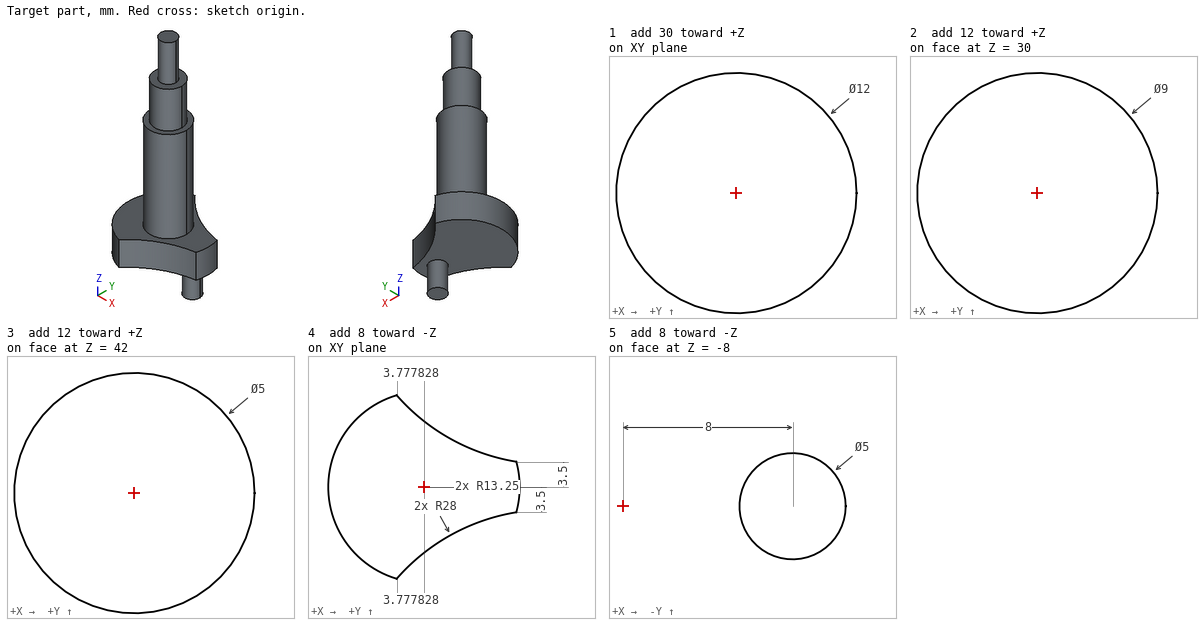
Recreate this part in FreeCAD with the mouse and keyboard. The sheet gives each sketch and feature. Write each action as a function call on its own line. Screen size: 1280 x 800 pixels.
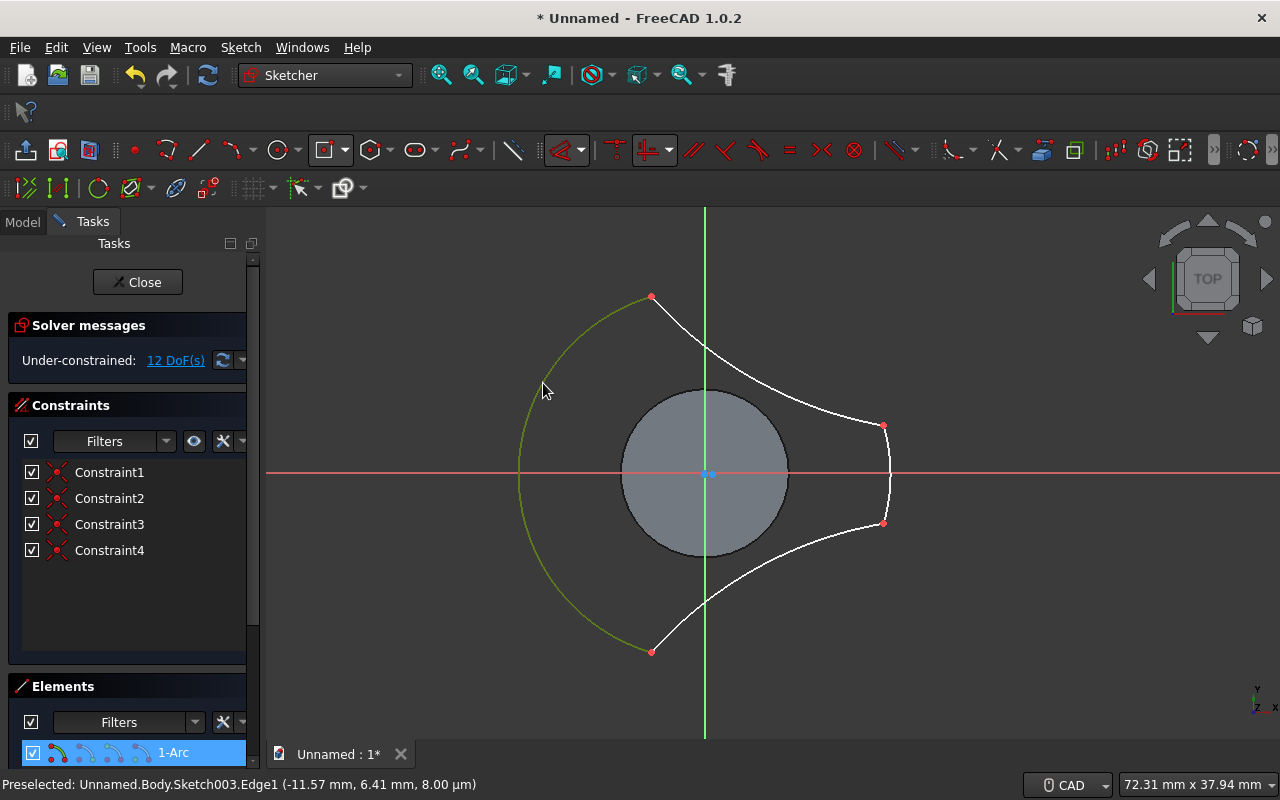
click(889, 494)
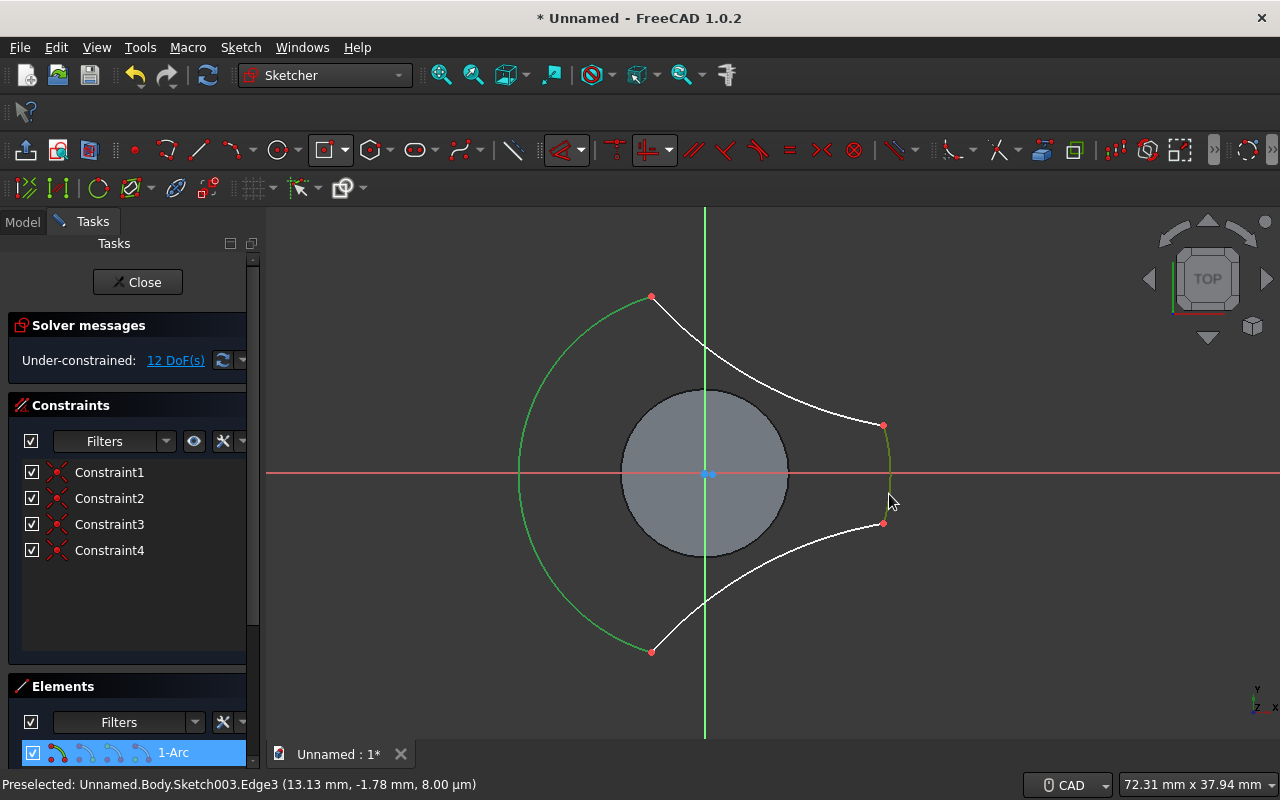
click(616, 150)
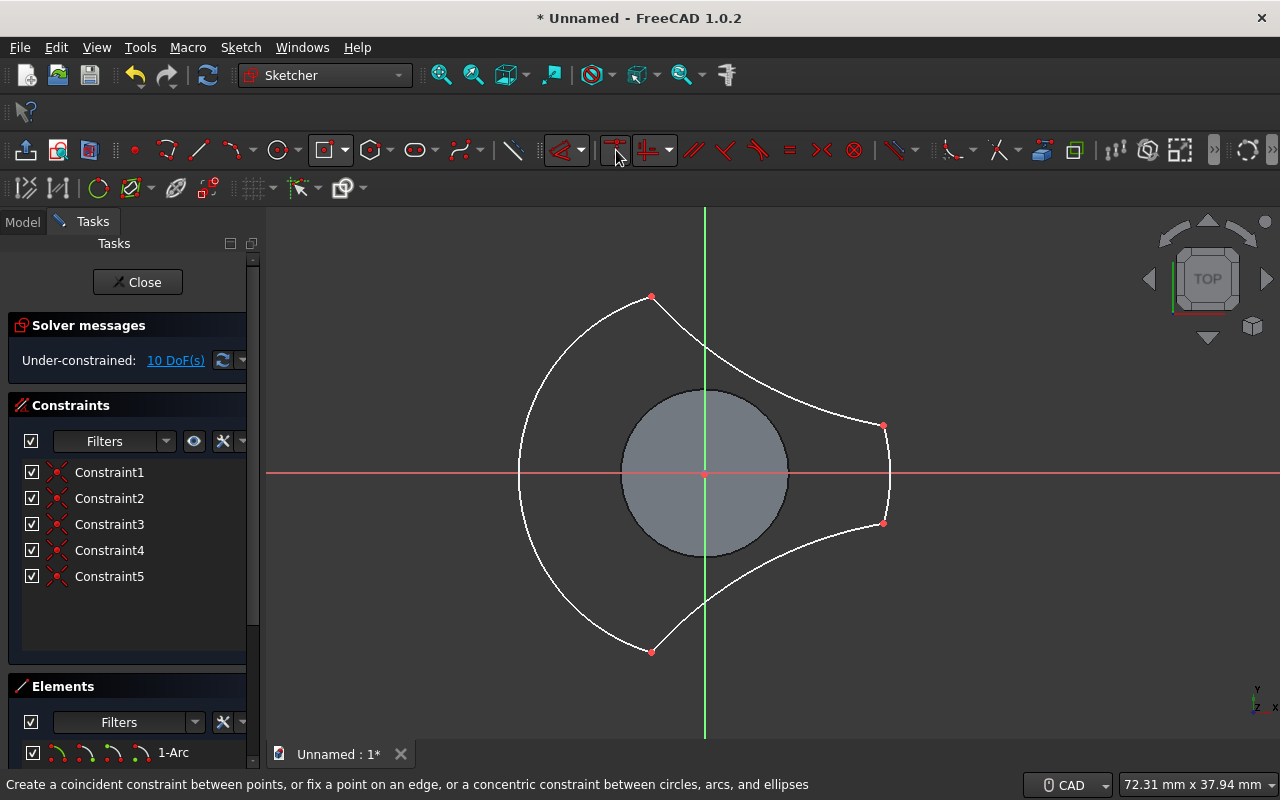
drag(694, 463, 715, 485)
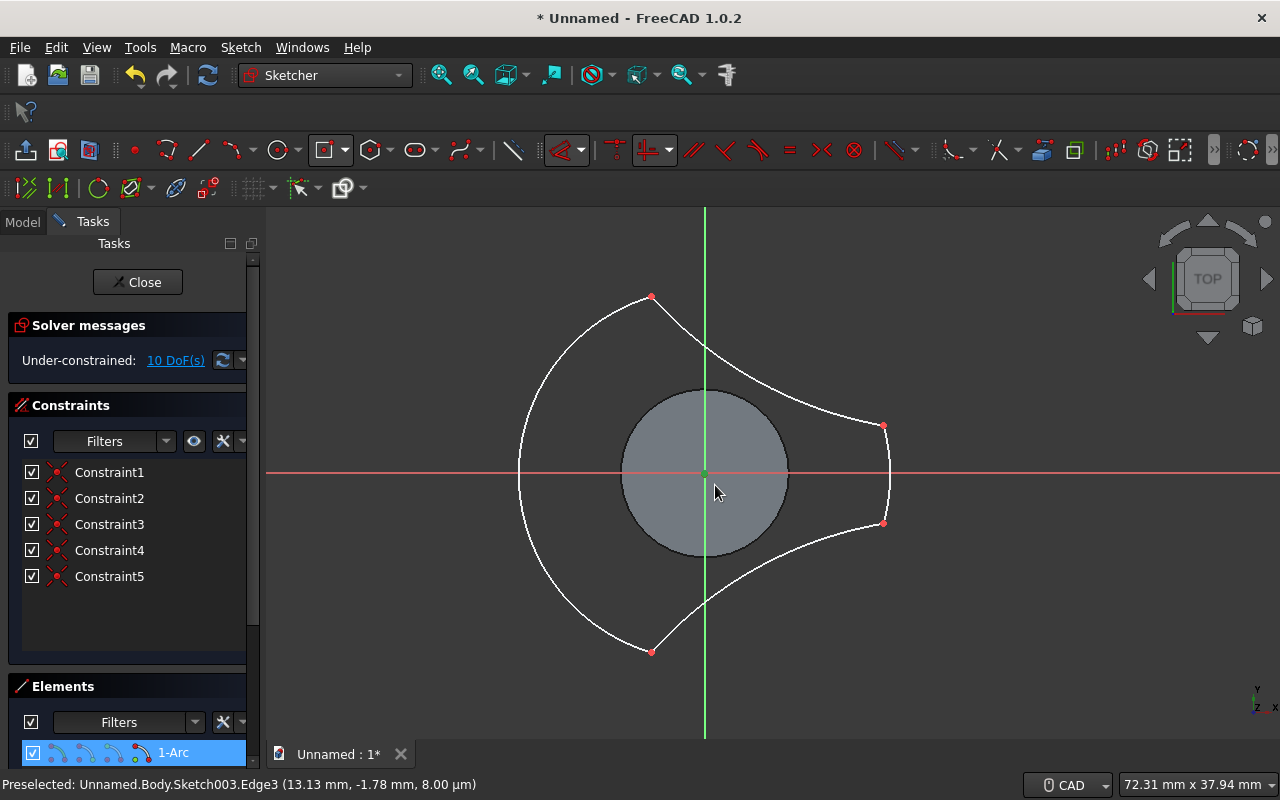
click(616, 150)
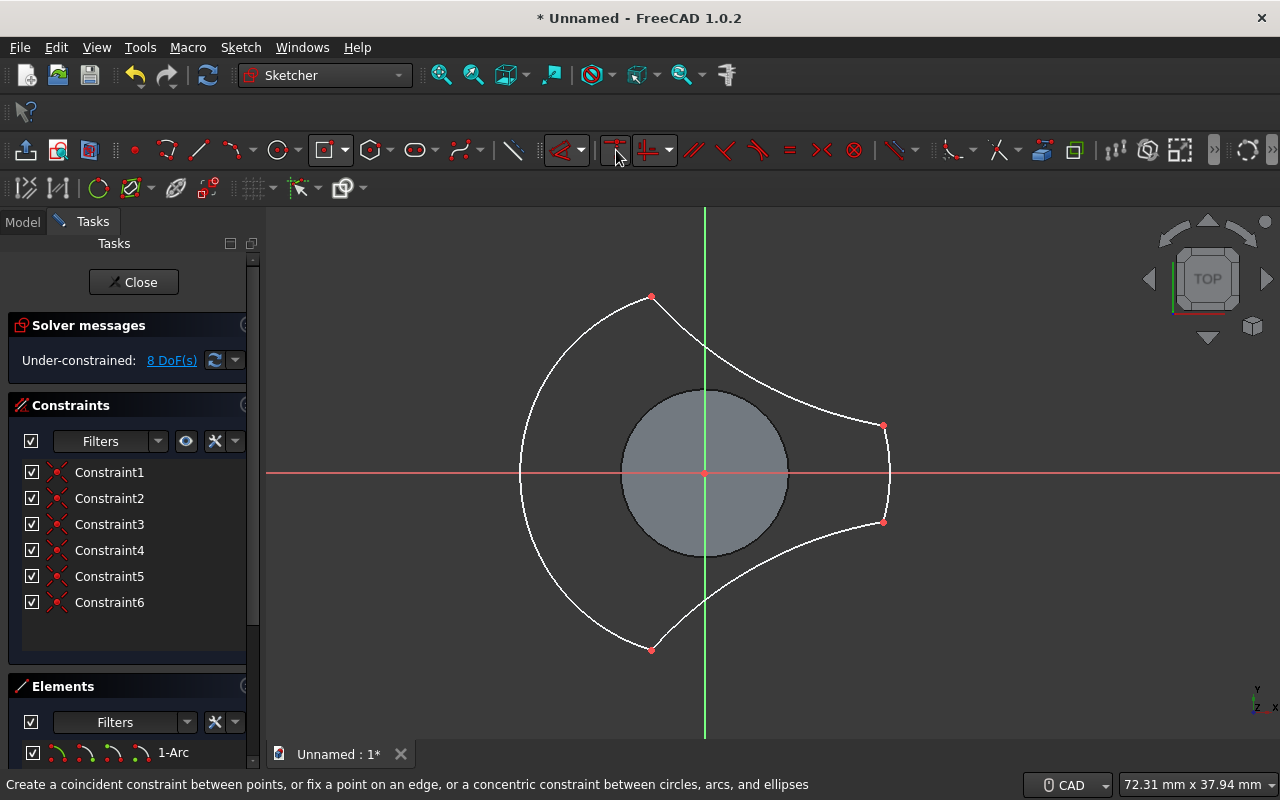
click(544, 383)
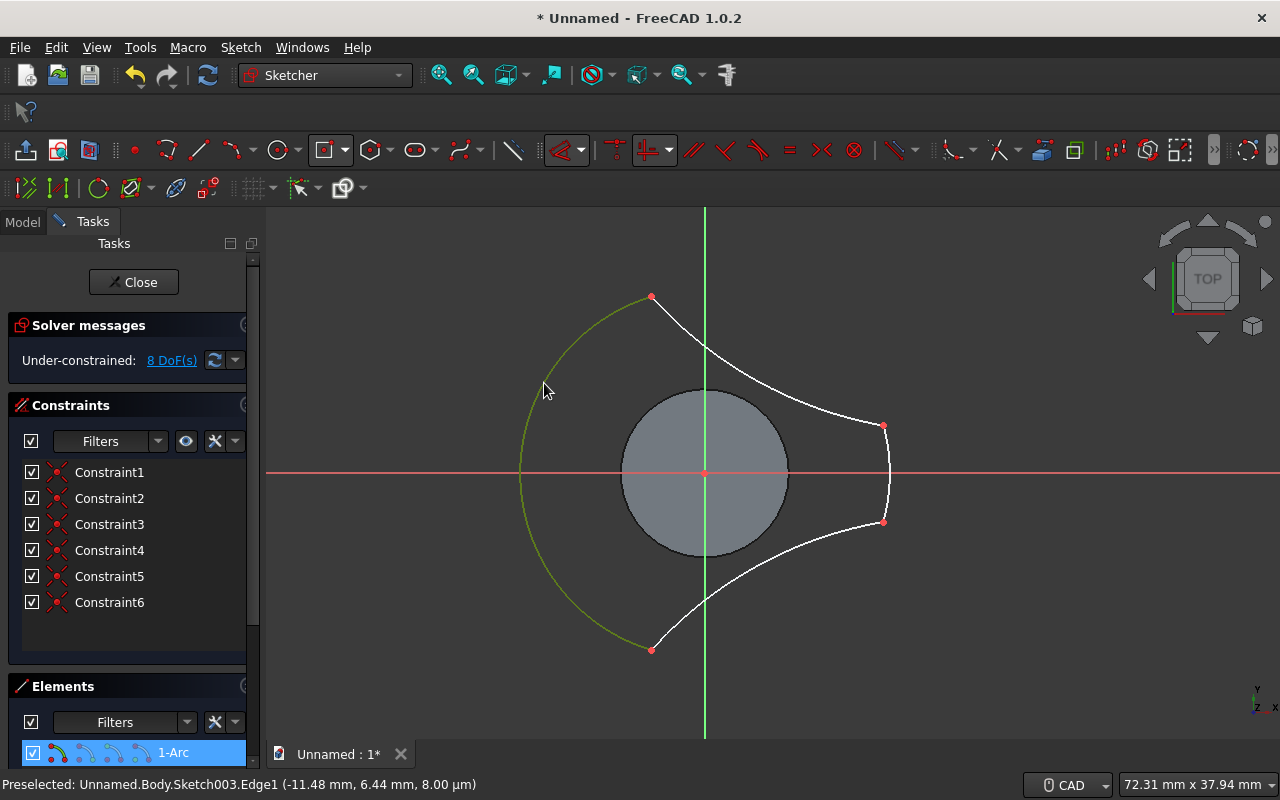
click(889, 493)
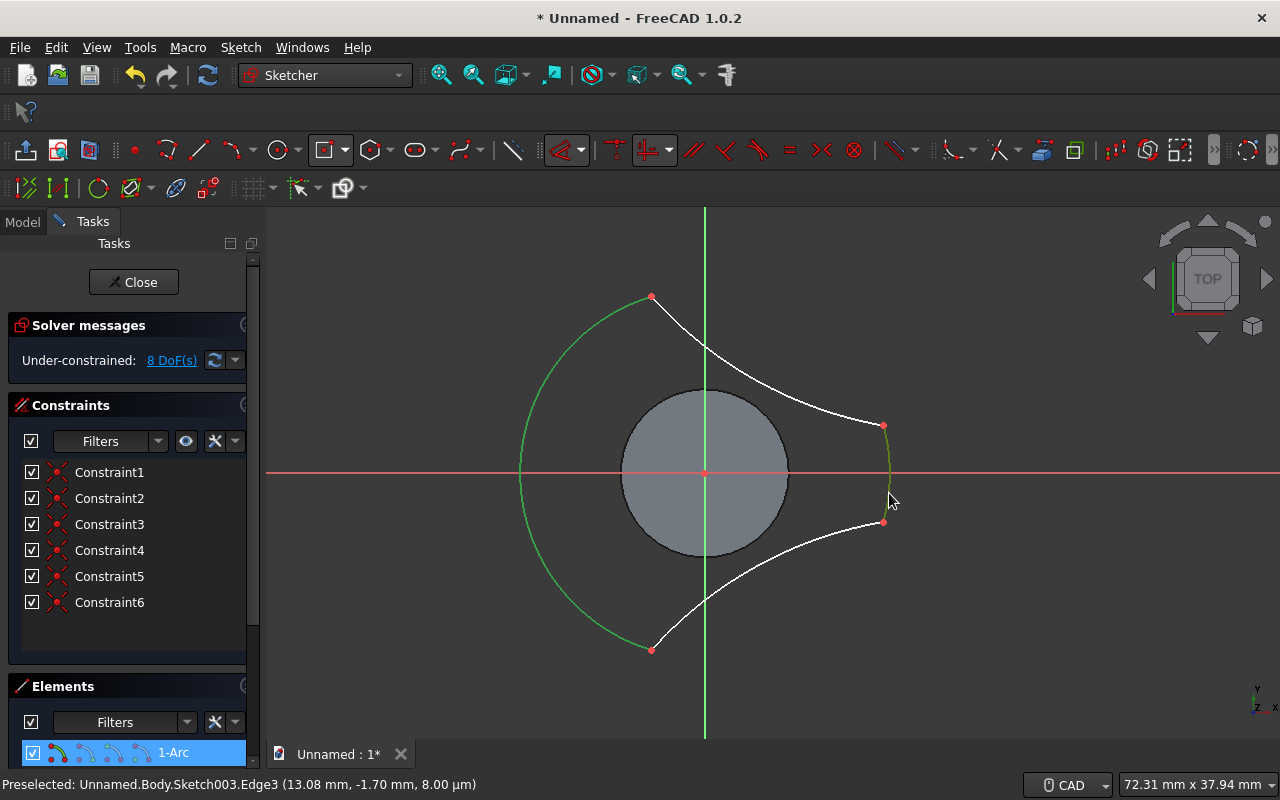
click(790, 150)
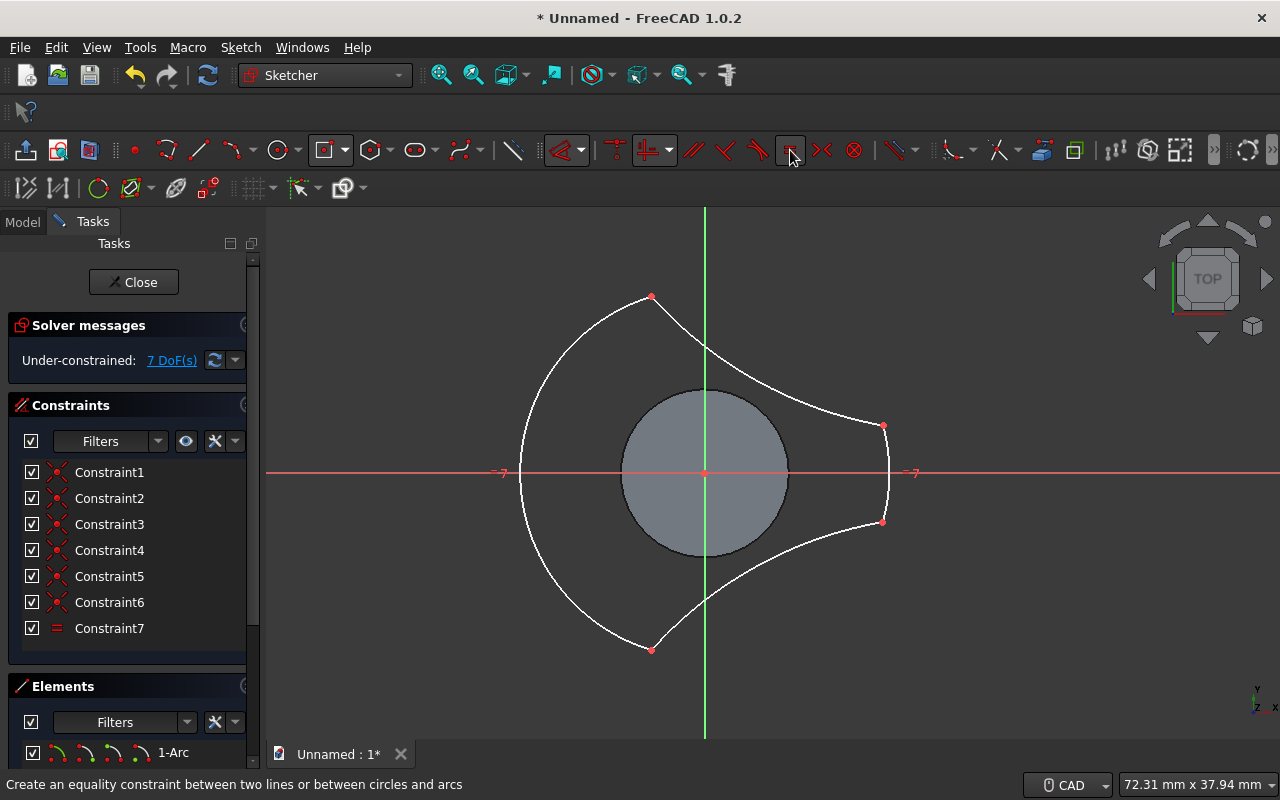
click(805, 404)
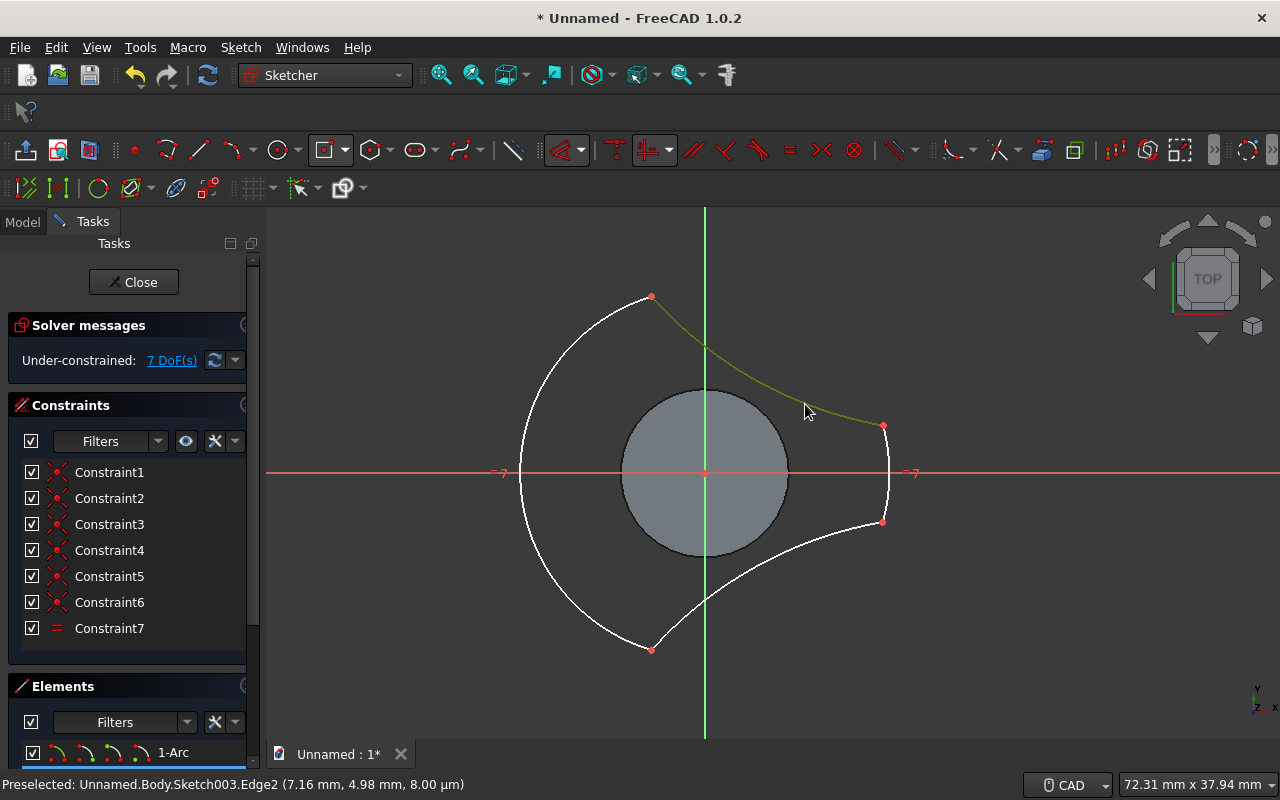
click(805, 544)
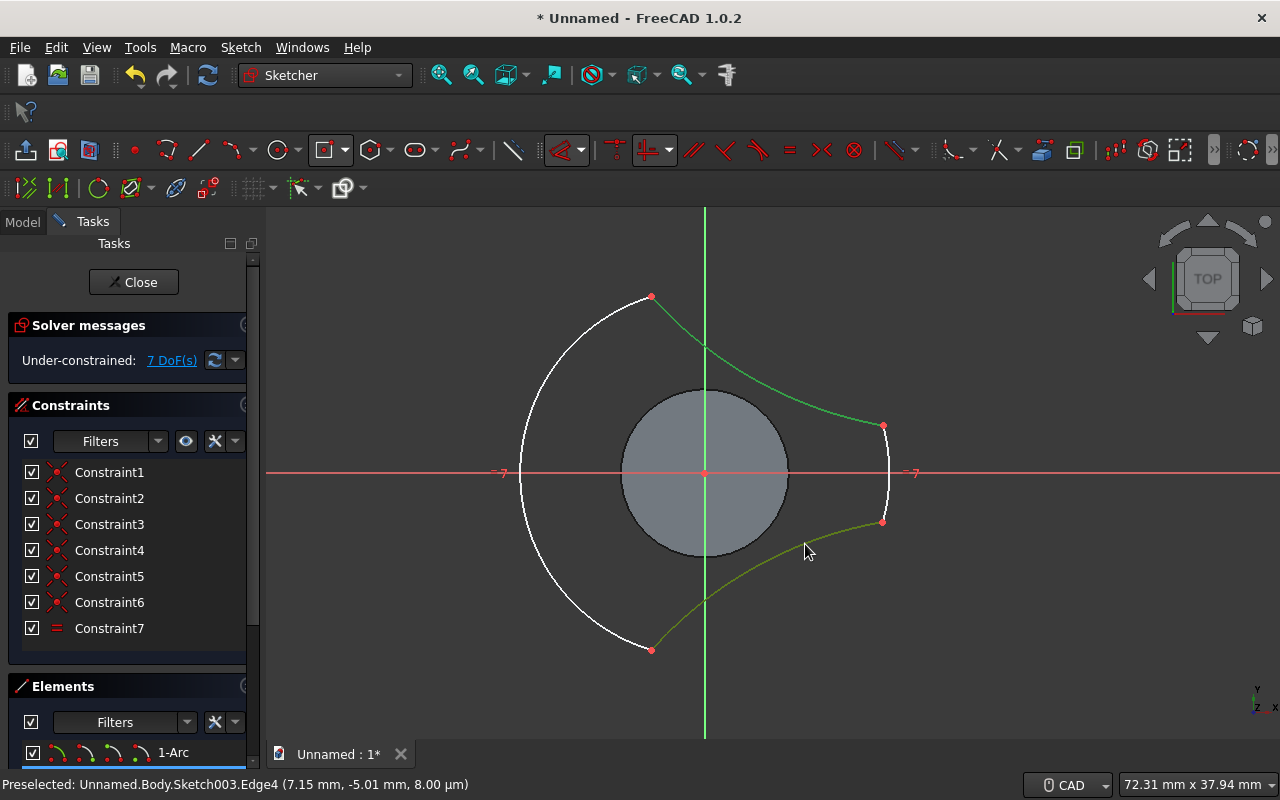
click(790, 150)